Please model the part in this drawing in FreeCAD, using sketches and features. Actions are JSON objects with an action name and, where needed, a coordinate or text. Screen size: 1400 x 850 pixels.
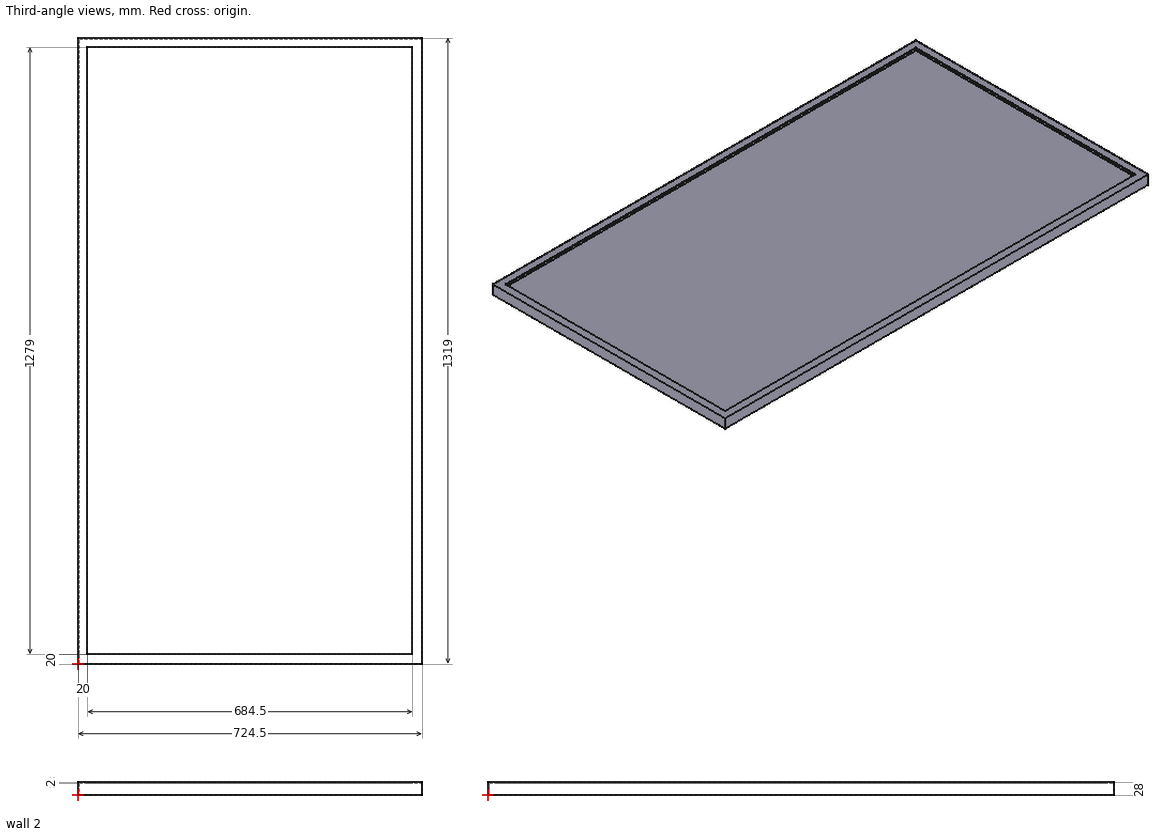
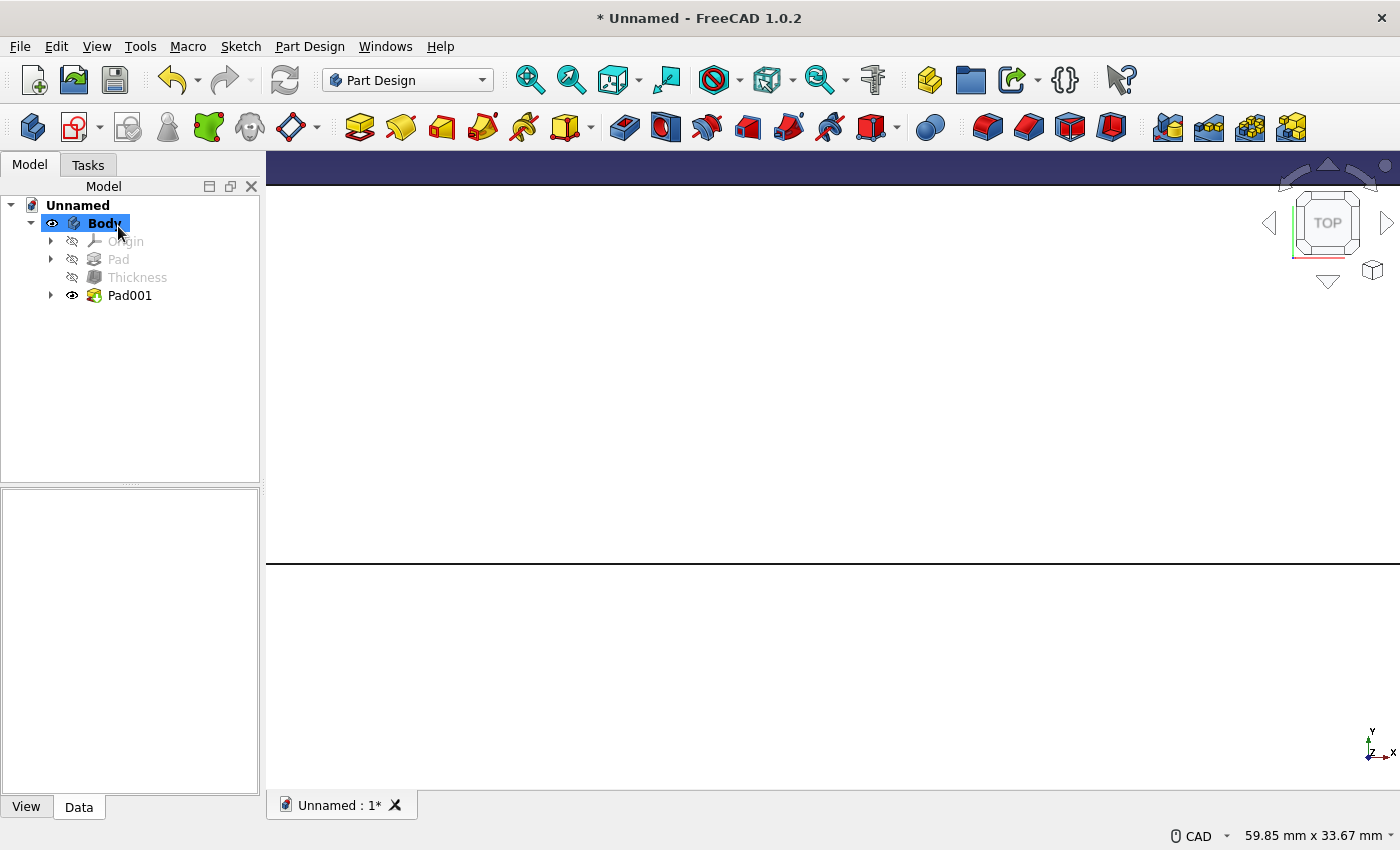
{"action": "key", "text": "0"}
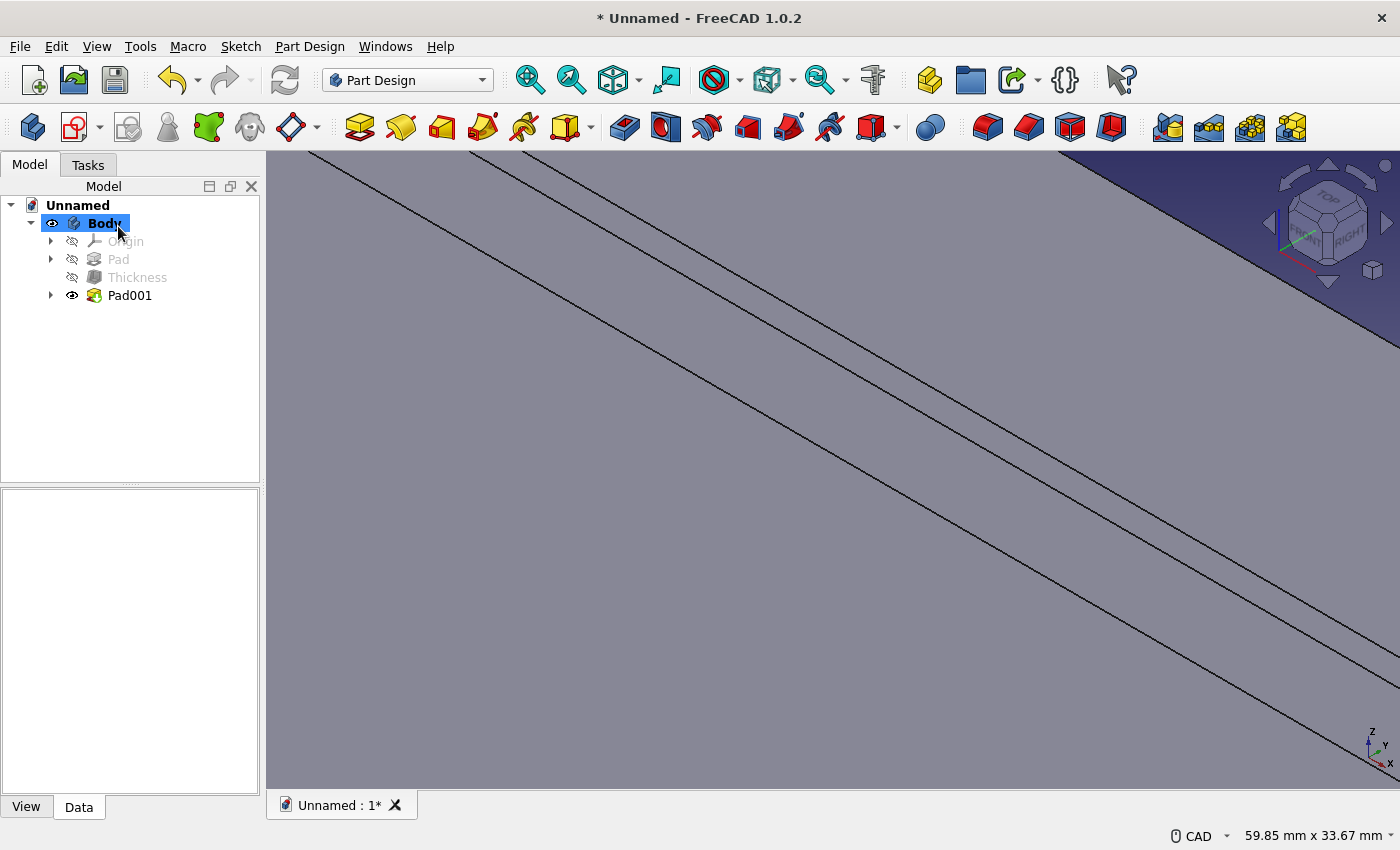
{"action": "left_click", "coordinate": [531, 80]}